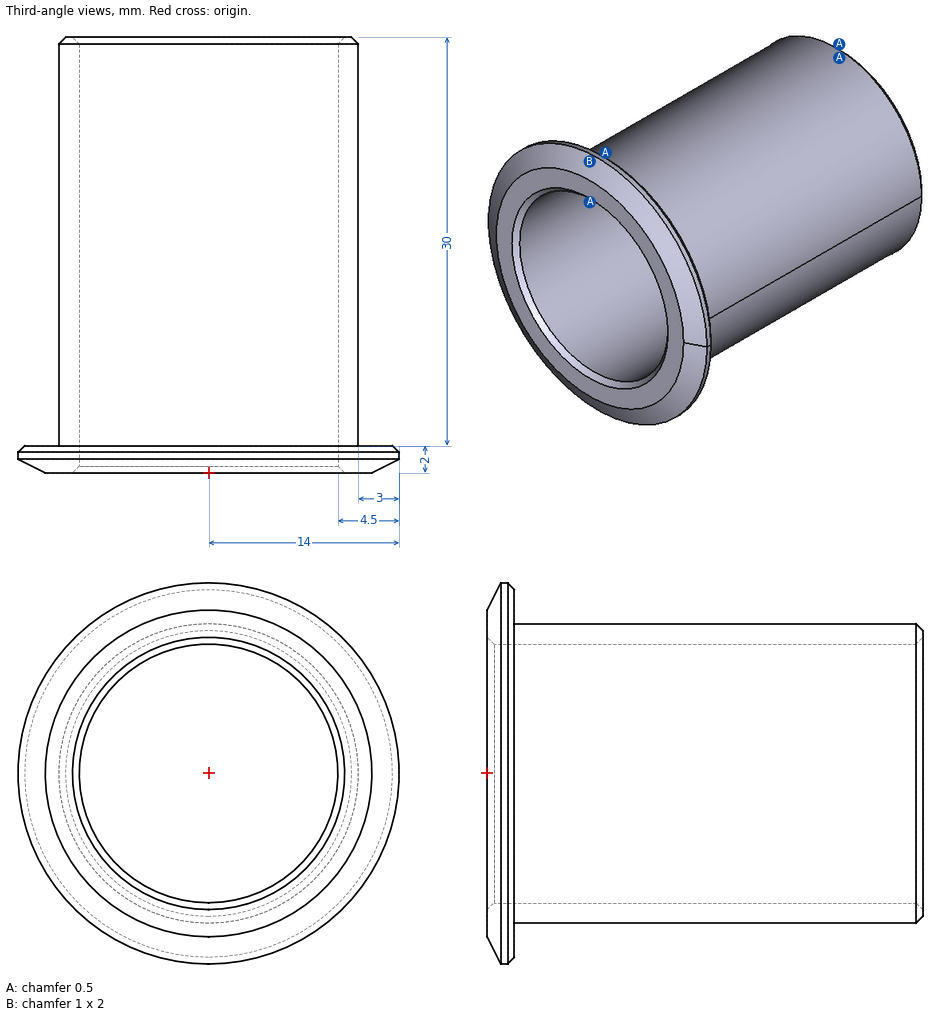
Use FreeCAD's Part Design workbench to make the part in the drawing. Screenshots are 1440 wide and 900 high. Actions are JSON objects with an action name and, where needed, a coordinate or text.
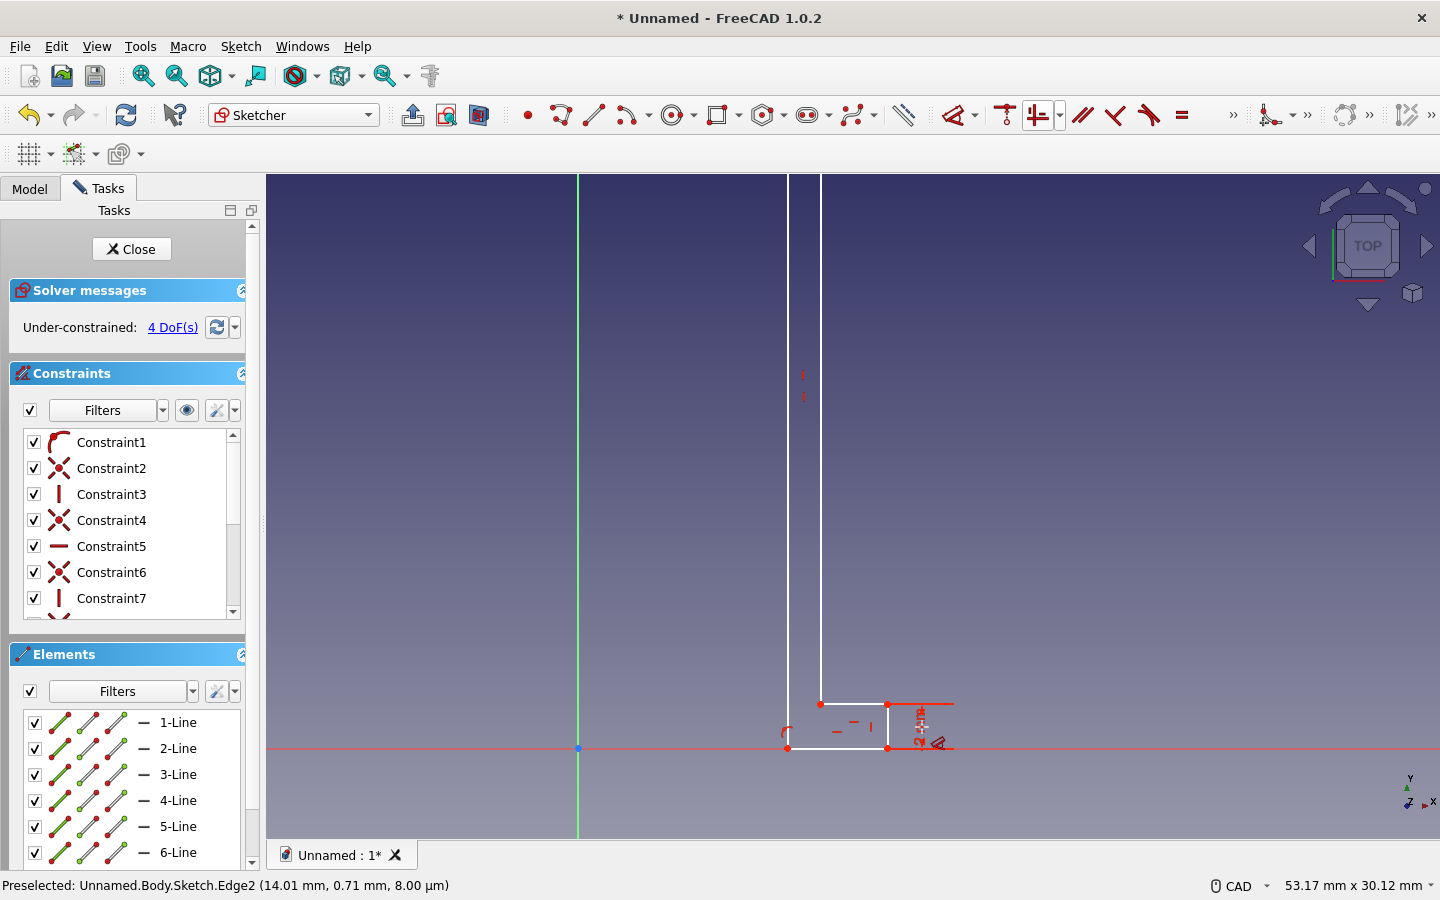
{"action": "left_click", "coordinate": [868, 704]}
{"action": "left_click", "coordinate": [854, 670]}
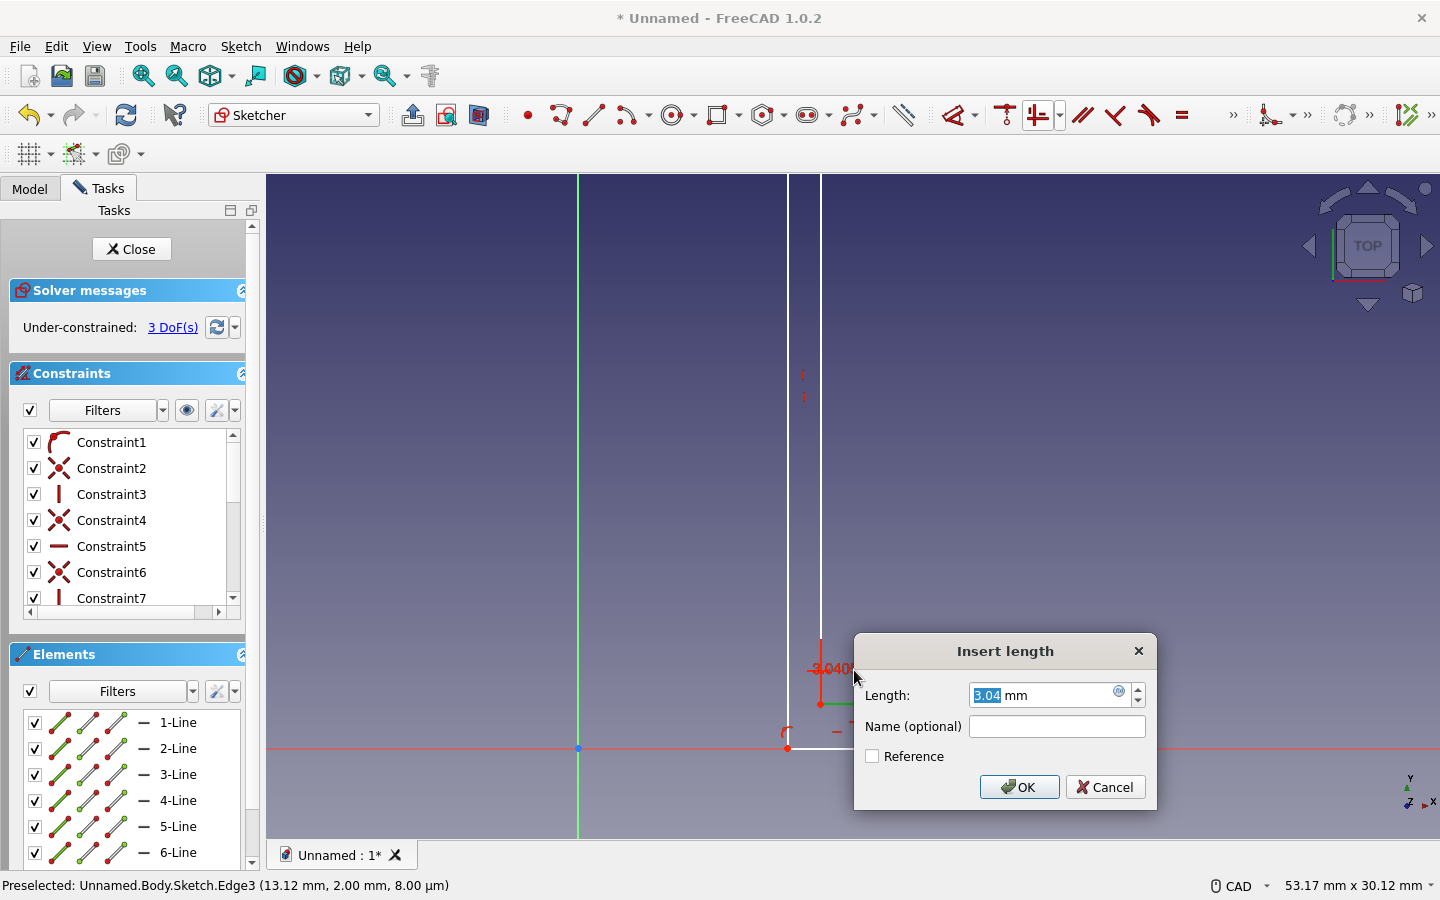
{"action": "type", "text": "3"}
{"action": "key", "text": "Return"}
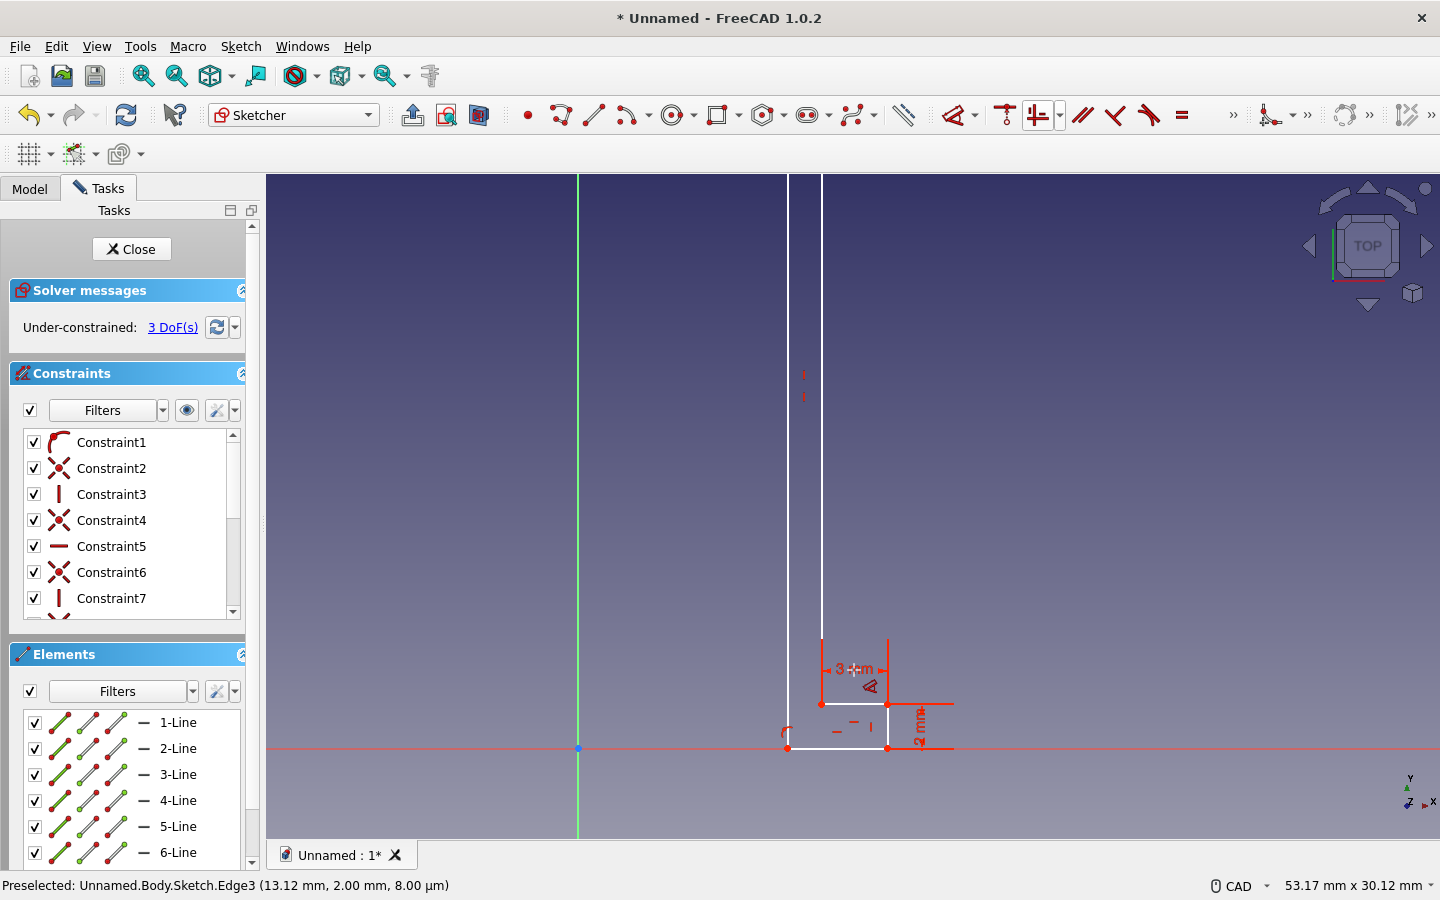
{"action": "left_click", "coordinate": [822, 506]}
{"action": "left_click", "coordinate": [856, 453]}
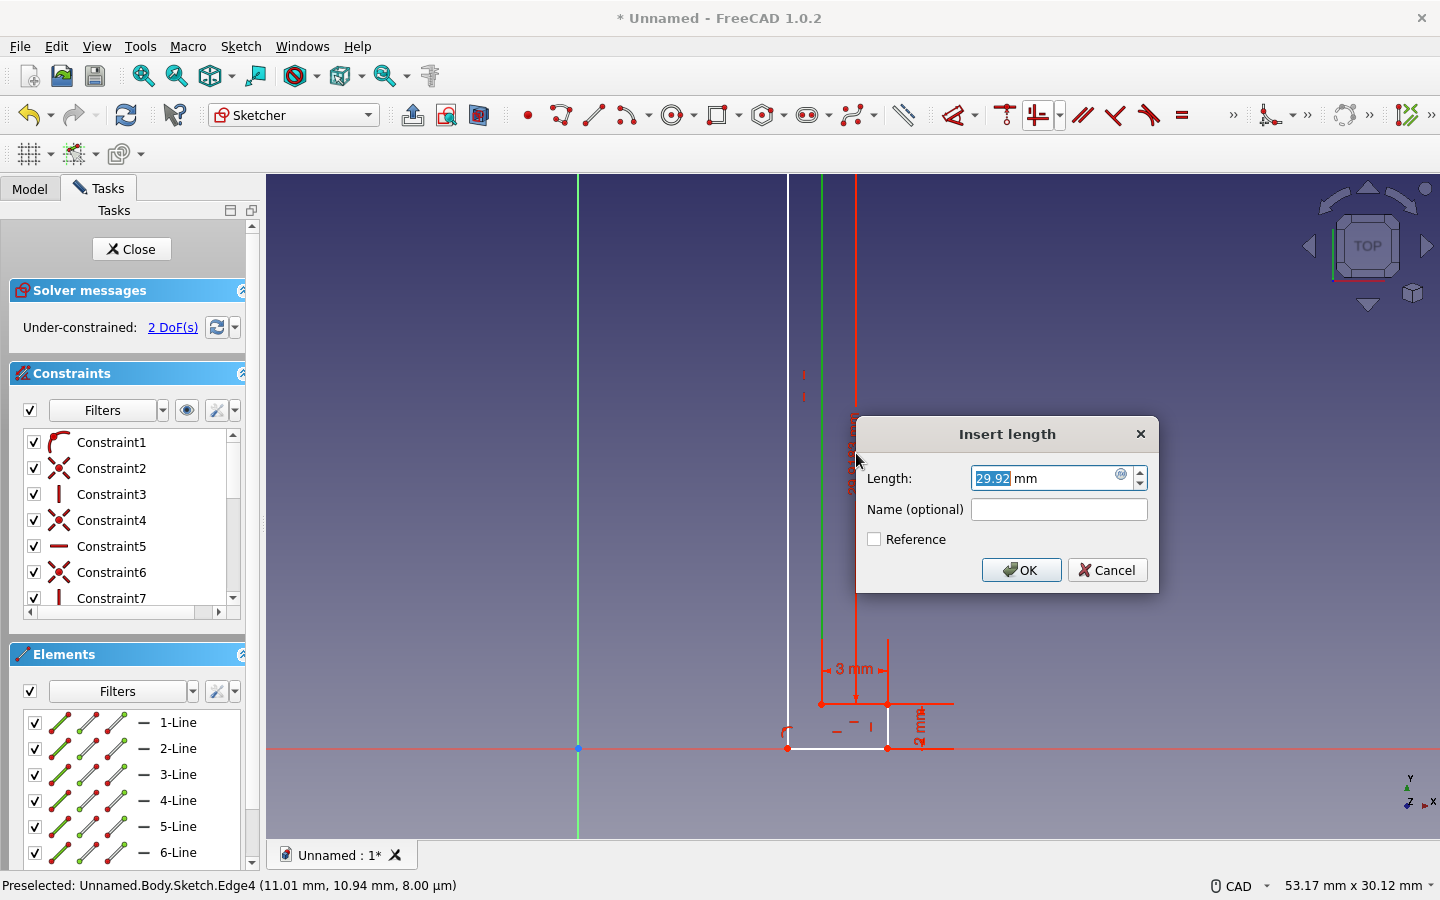
{"action": "type", "text": "30"}
{"action": "key", "text": "Return"}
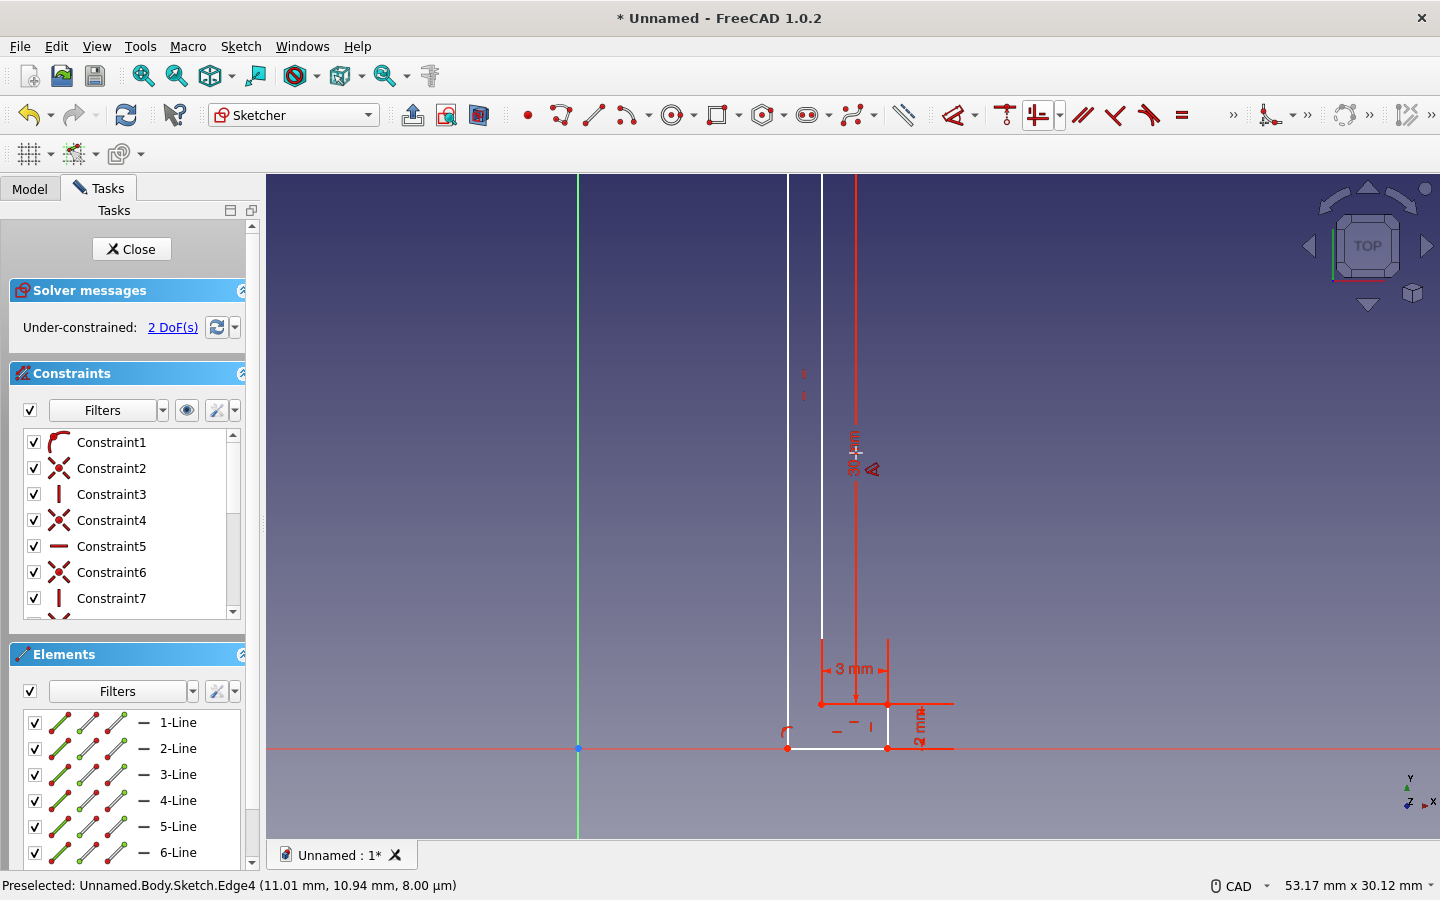
{"action": "left_click", "coordinate": [818, 749]}
{"action": "left_click", "coordinate": [838, 783]}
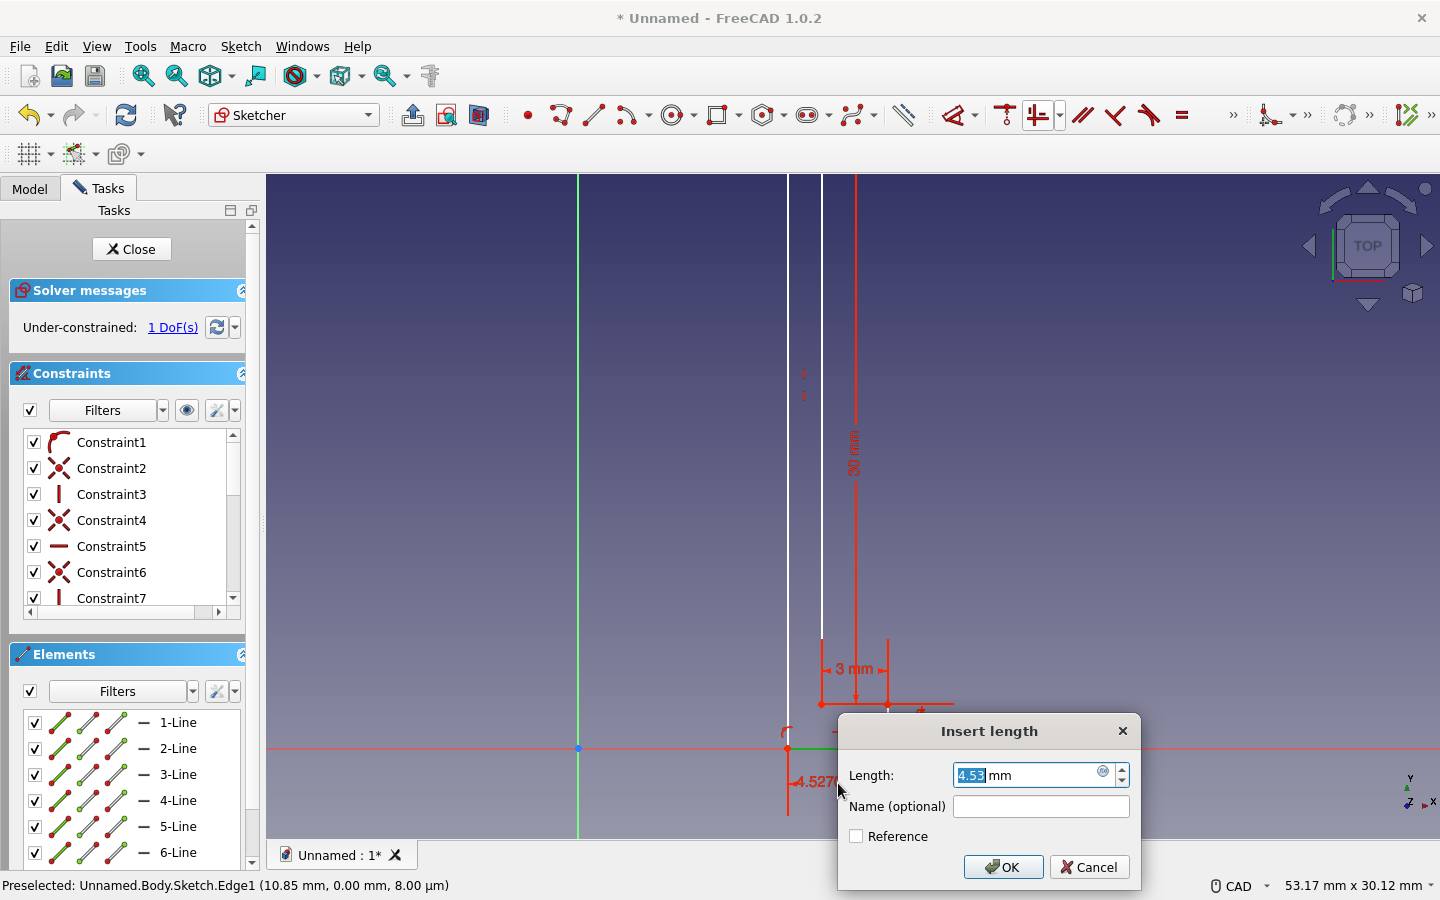
{"action": "type", "text": "4.5"}
{"action": "key", "text": "Return"}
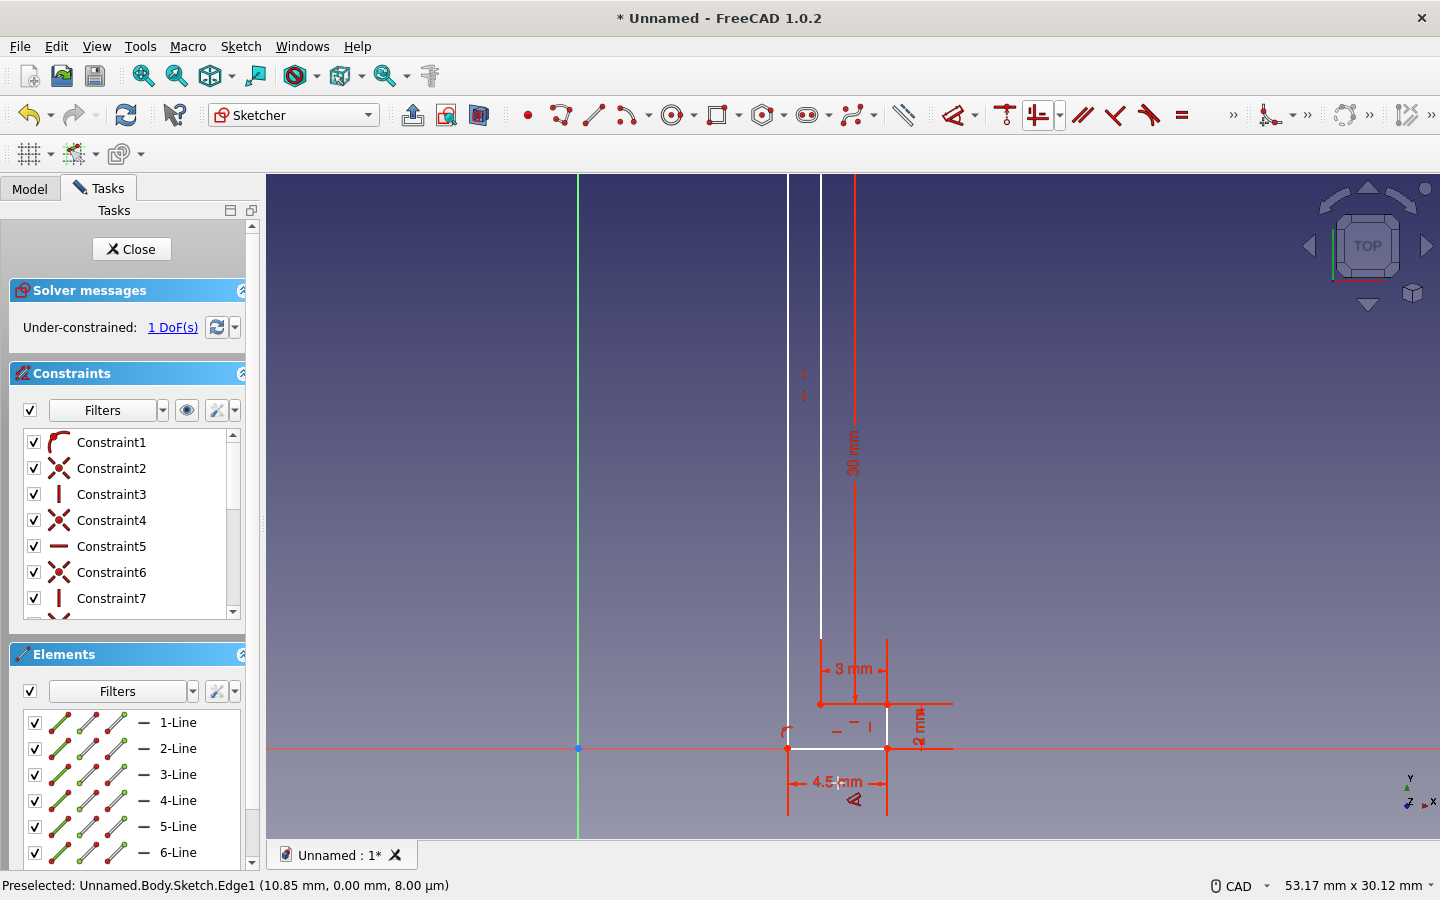
{"action": "left_click", "coordinate": [887, 749]}
{"action": "left_click", "coordinate": [733, 783]}